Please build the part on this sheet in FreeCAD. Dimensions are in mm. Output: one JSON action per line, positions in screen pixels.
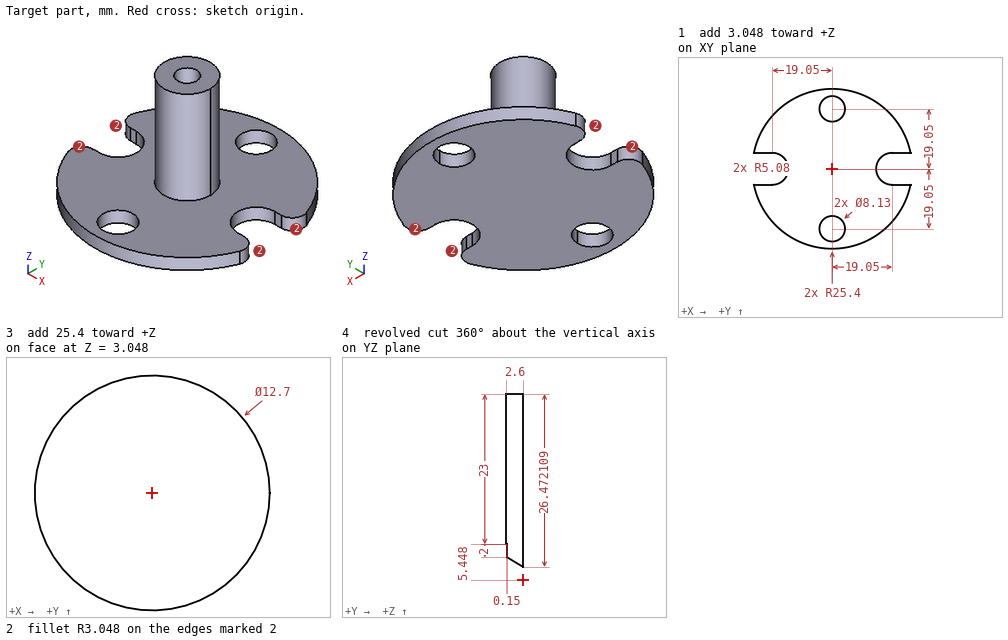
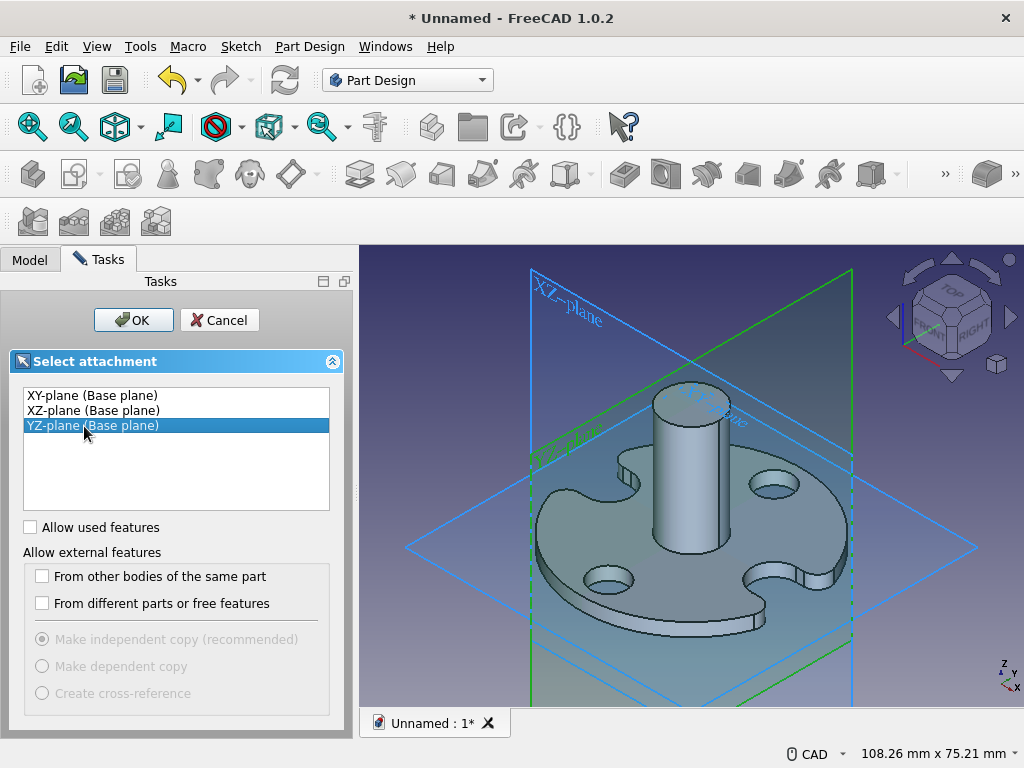
{"action": "left_click", "coordinate": [134, 320]}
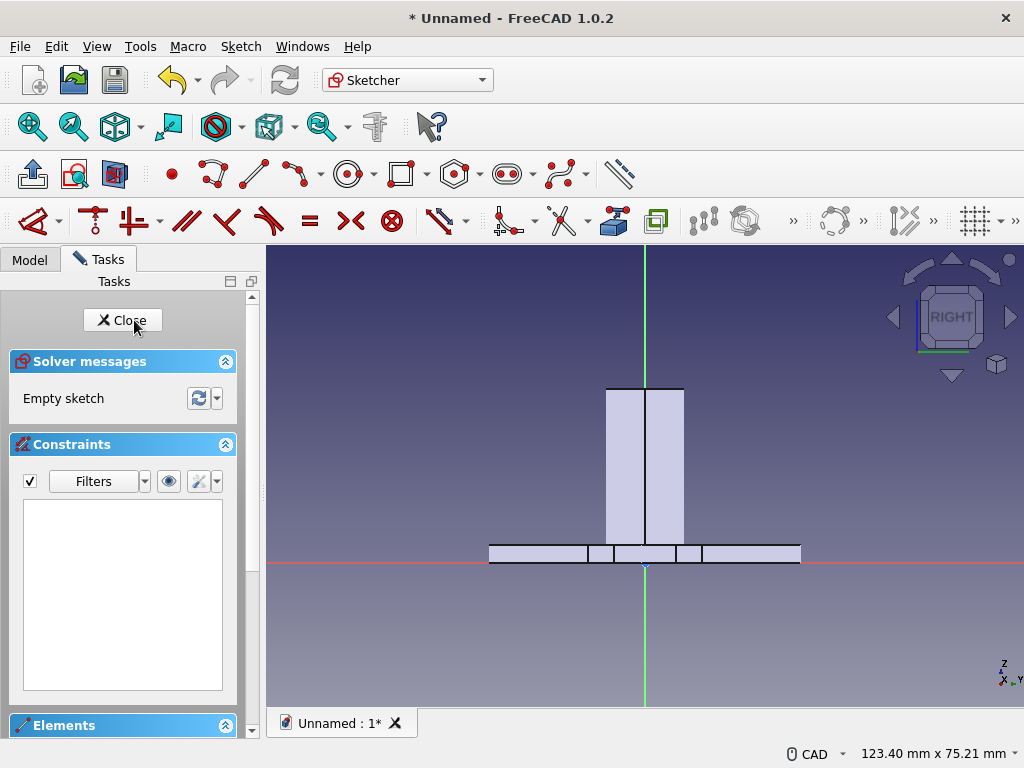
{"action": "left_click", "coordinate": [115, 174]}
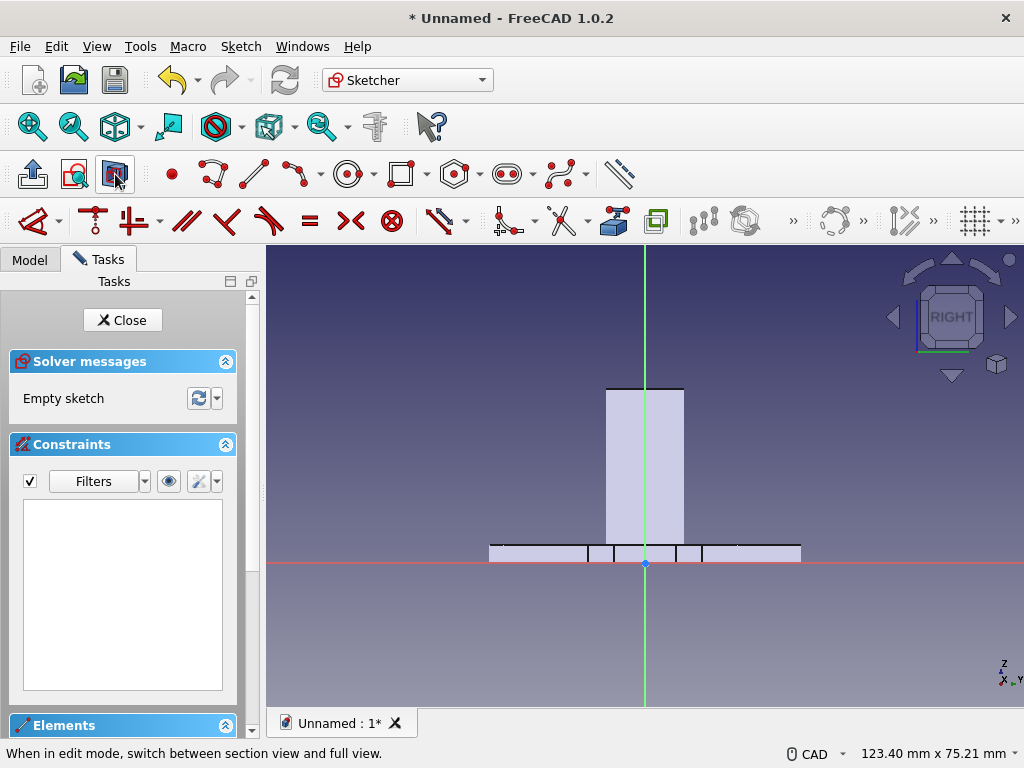
{"action": "scroll", "coordinate": [760, 476], "scroll_direction": "up", "scroll_amount": 2}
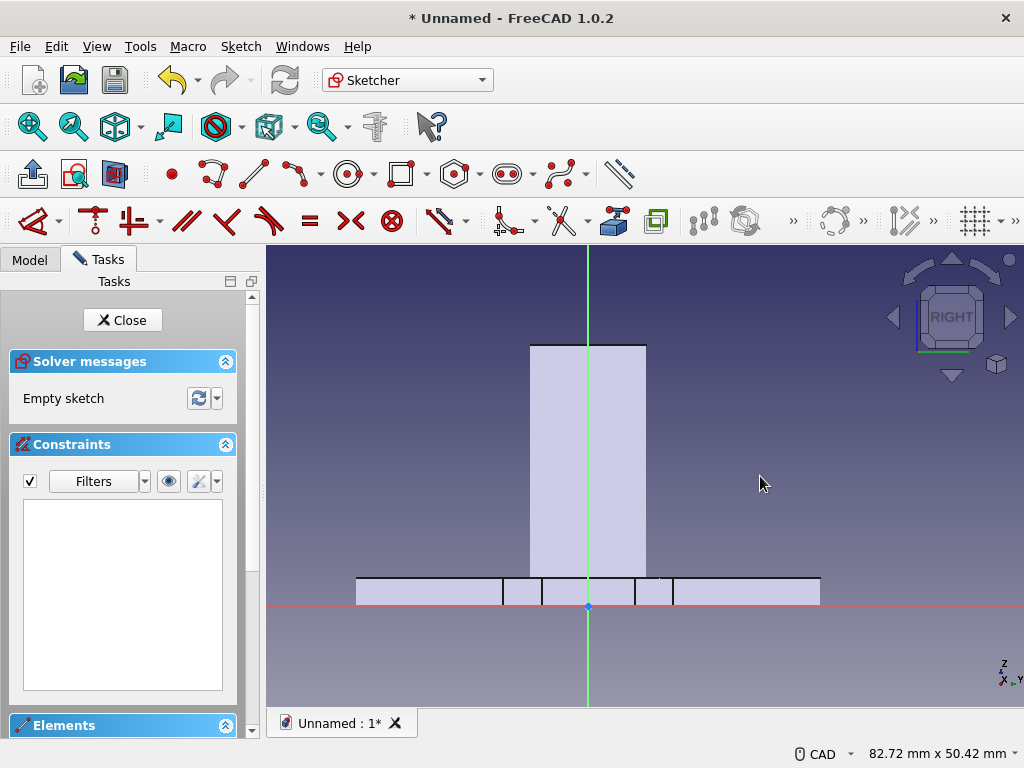
{"action": "left_click", "coordinate": [213, 174]}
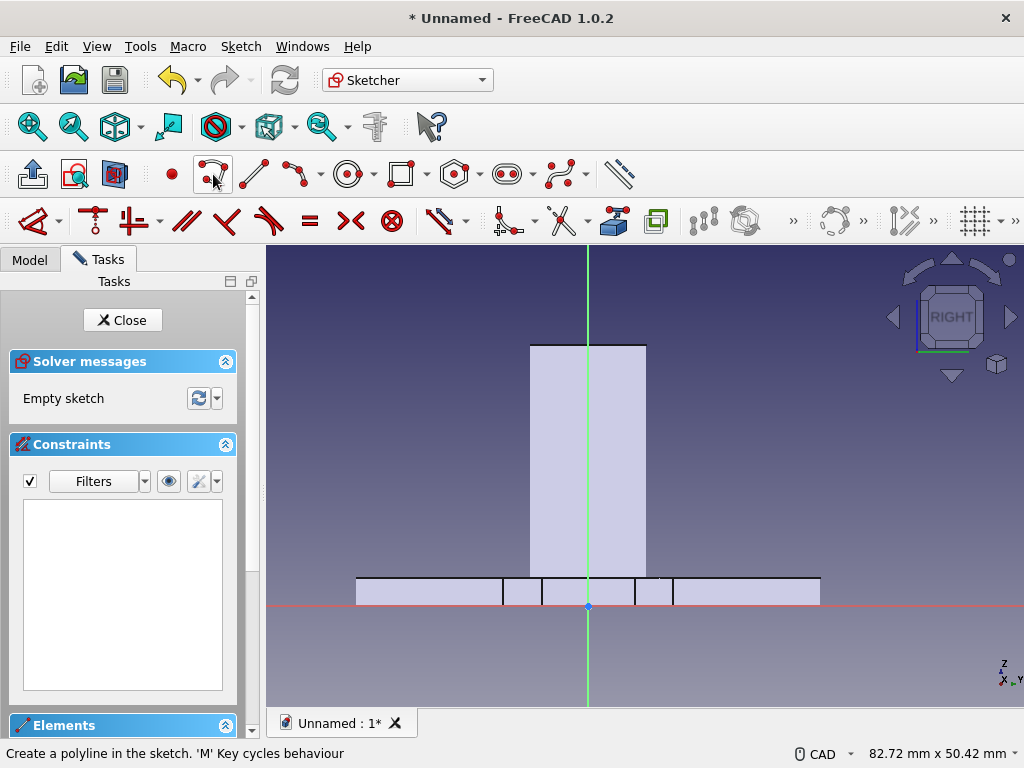
{"action": "left_click", "coordinate": [588, 588]}
{"action": "left_click", "coordinate": [579, 345]}
{"action": "left_click", "coordinate": [564, 345]}
{"action": "left_click", "coordinate": [564, 556]}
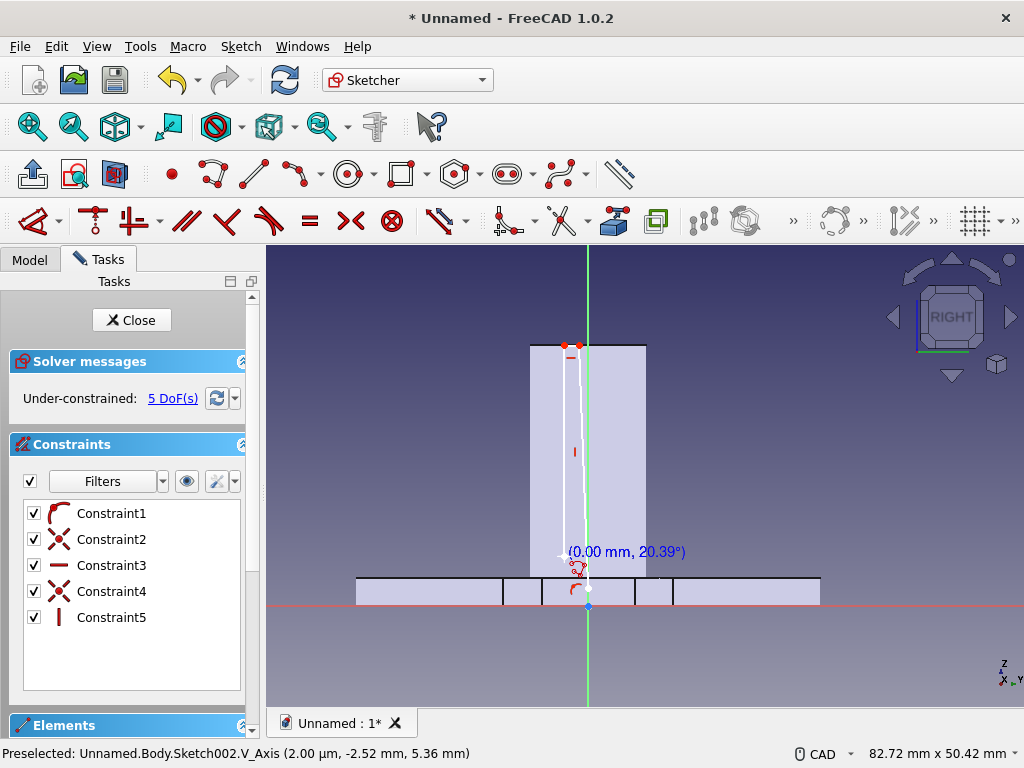
{"action": "scroll", "coordinate": [566, 556], "scroll_direction": "up", "scroll_amount": 13}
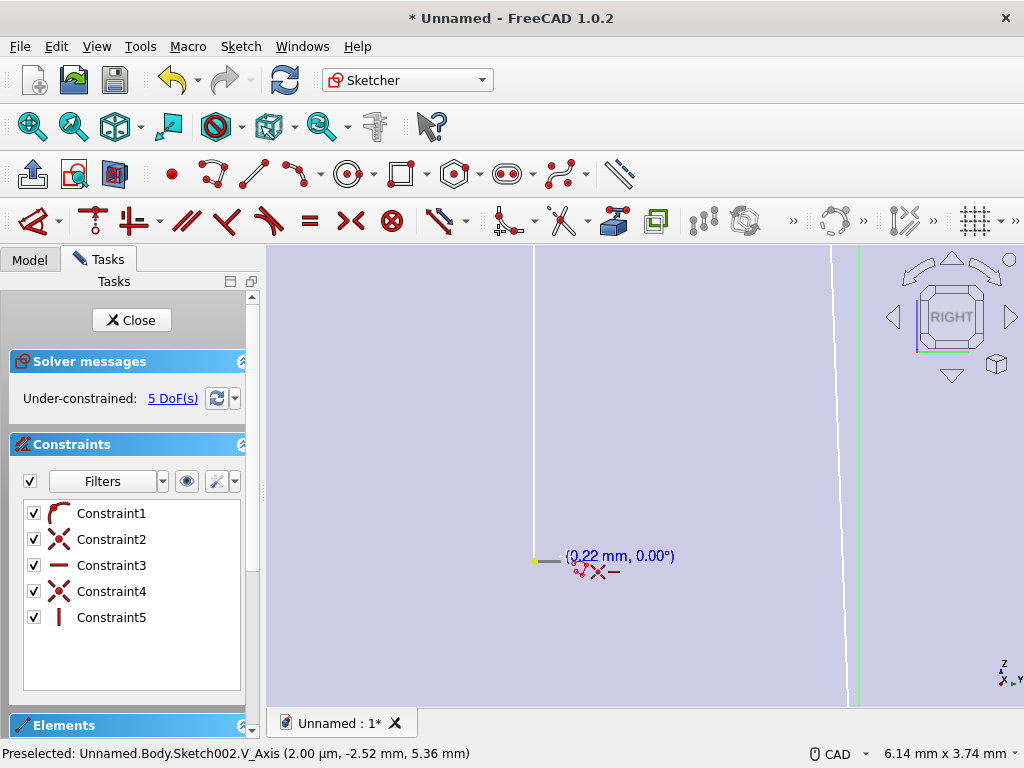
{"action": "left_click", "coordinate": [557, 548]}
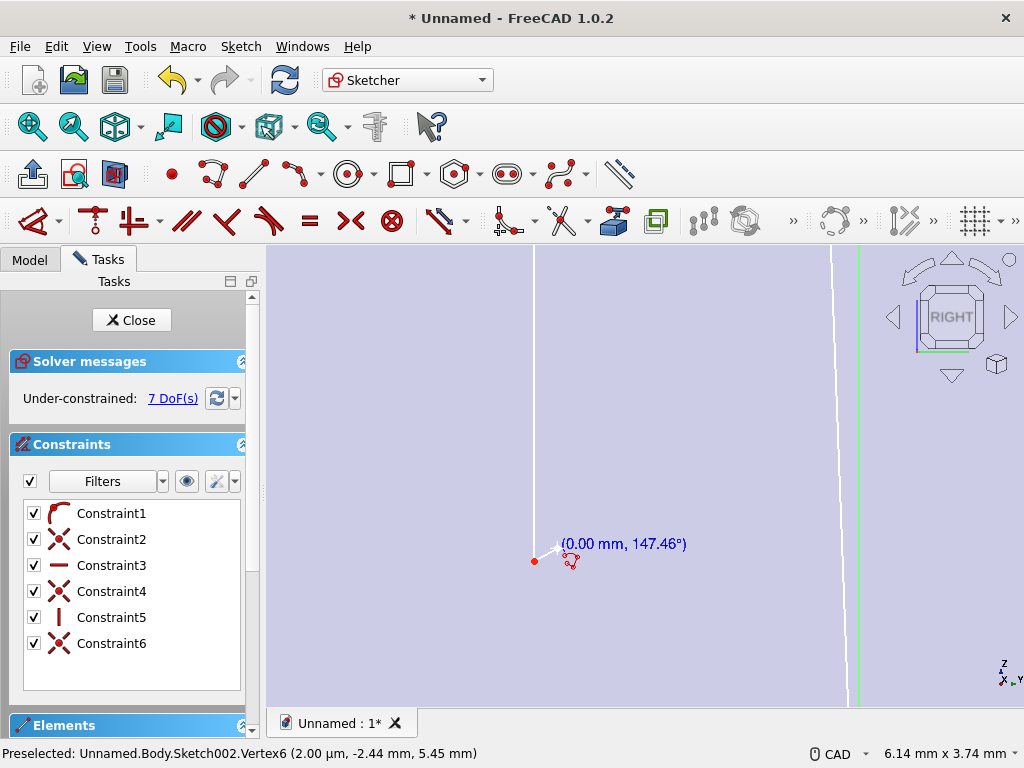
{"action": "scroll", "coordinate": [567, 557], "scroll_direction": "down", "scroll_amount": 13}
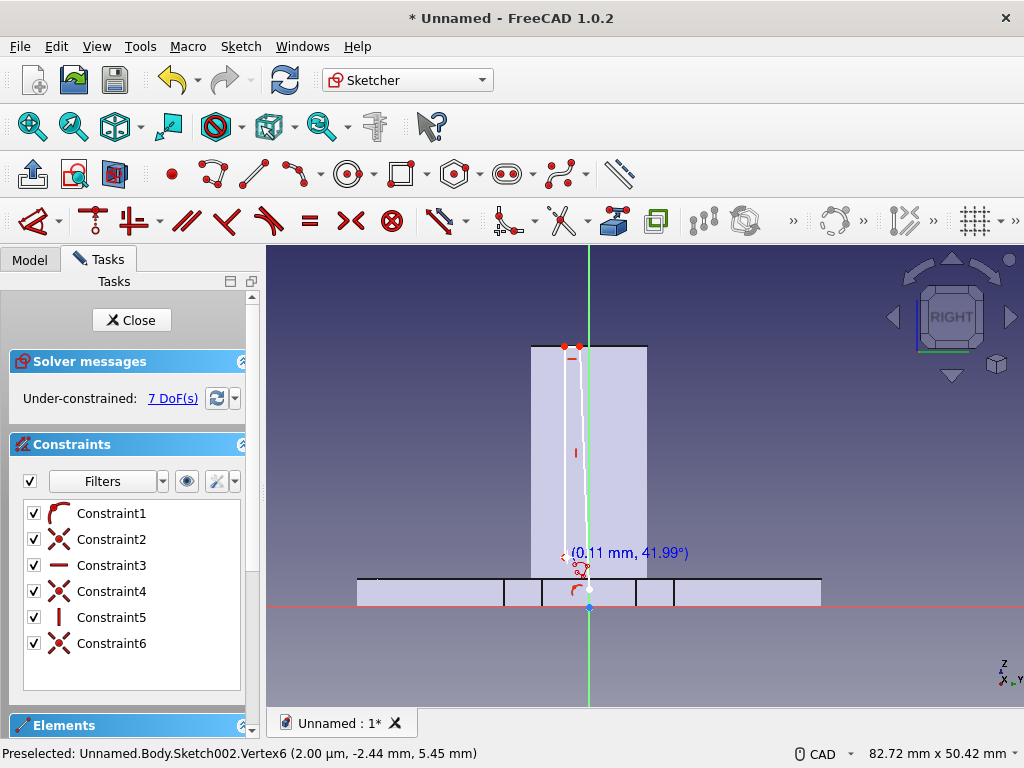
{"action": "left_click", "coordinate": [567, 575]}
{"action": "left_click", "coordinate": [589, 590]}
{"action": "key", "text": "Escape"}
{"action": "key", "text": "Escape"}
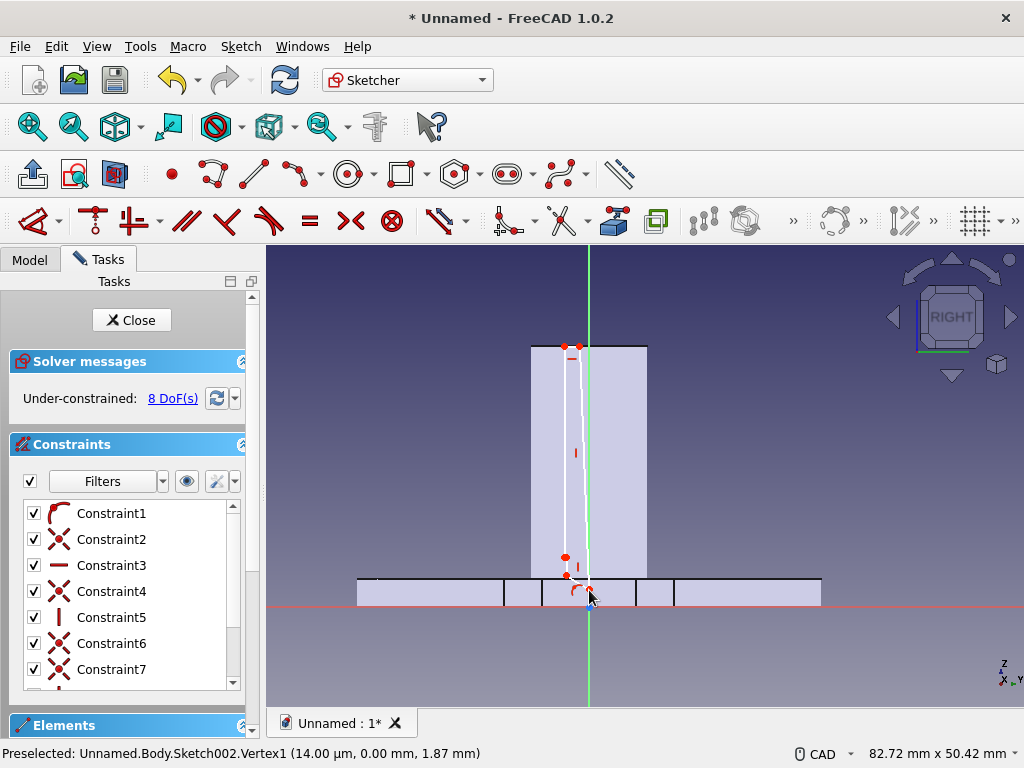
{"action": "left_click", "coordinate": [586, 517]}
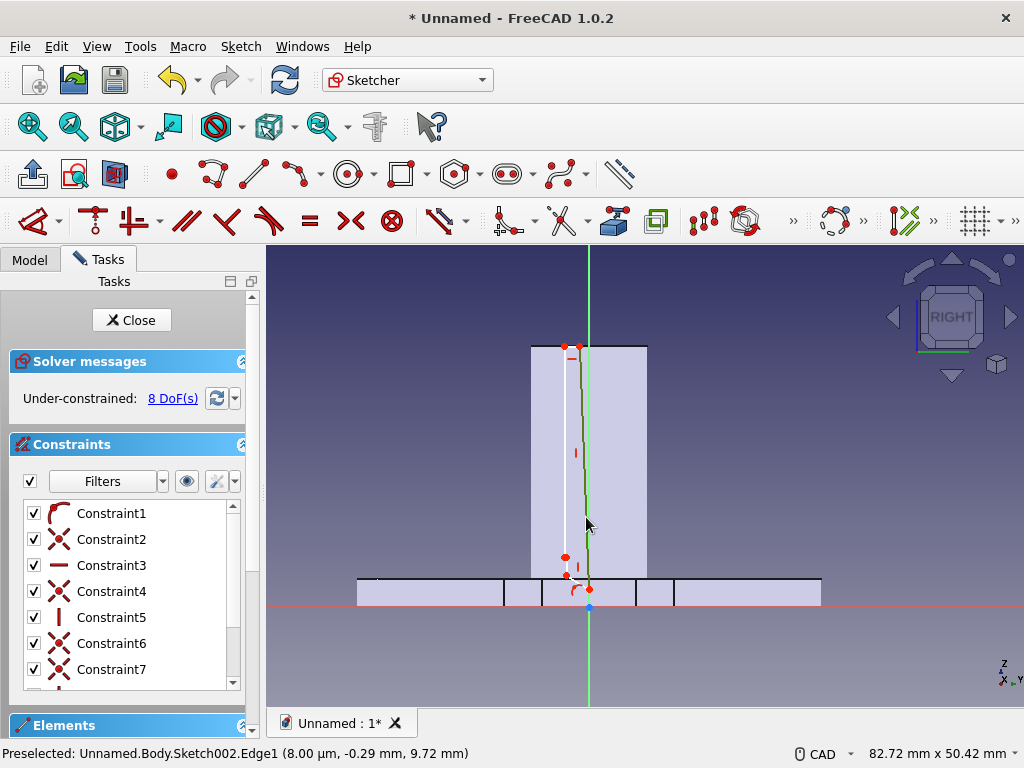
{"action": "left_click", "coordinate": [160, 222]}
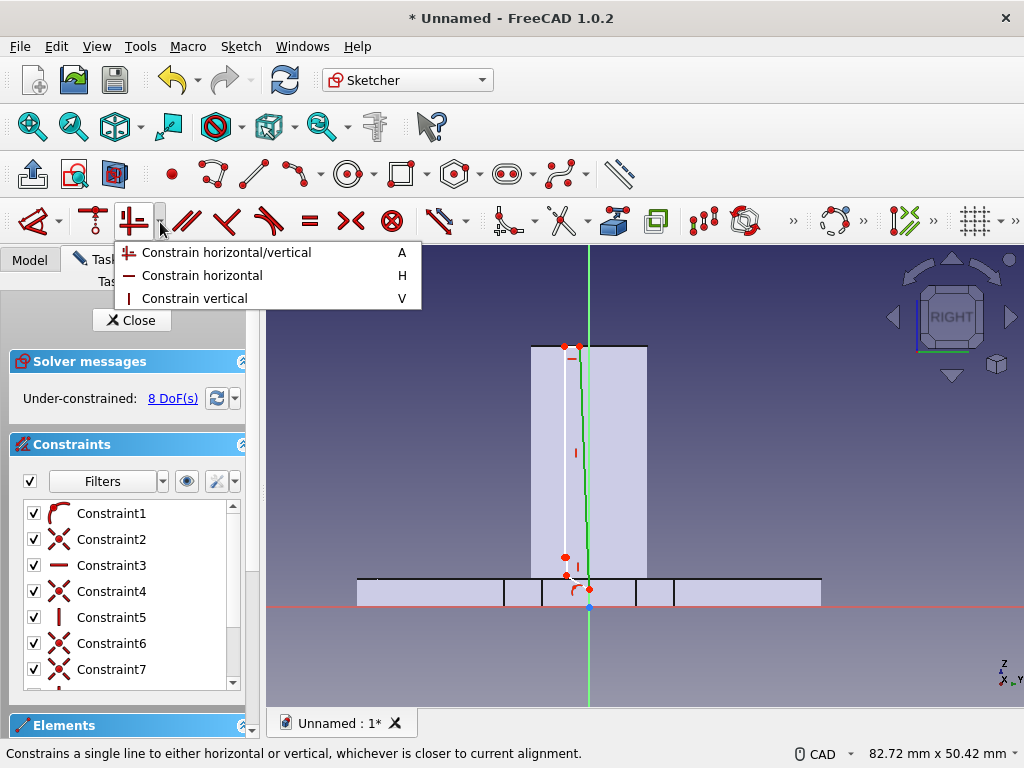
{"action": "left_click", "coordinate": [268, 298]}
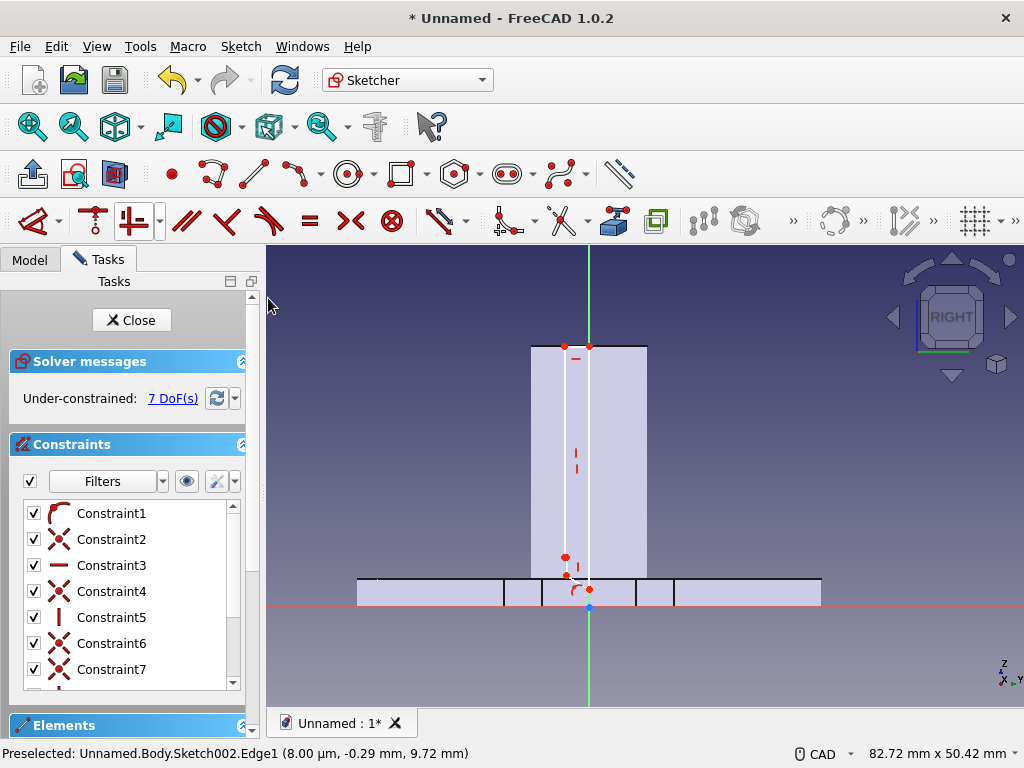
{"action": "scroll", "coordinate": [566, 557], "scroll_direction": "up", "scroll_amount": 14}